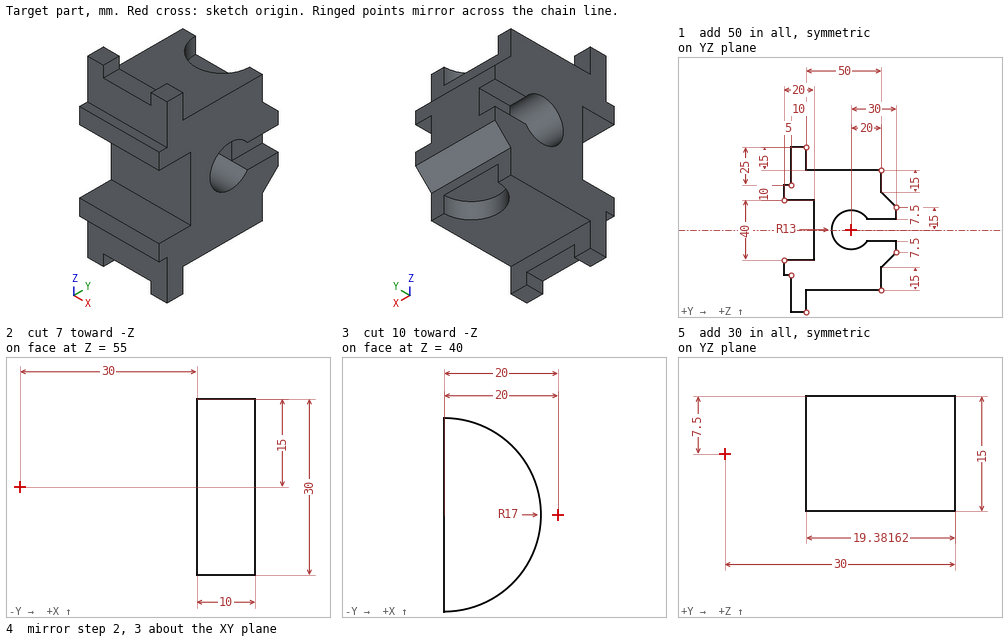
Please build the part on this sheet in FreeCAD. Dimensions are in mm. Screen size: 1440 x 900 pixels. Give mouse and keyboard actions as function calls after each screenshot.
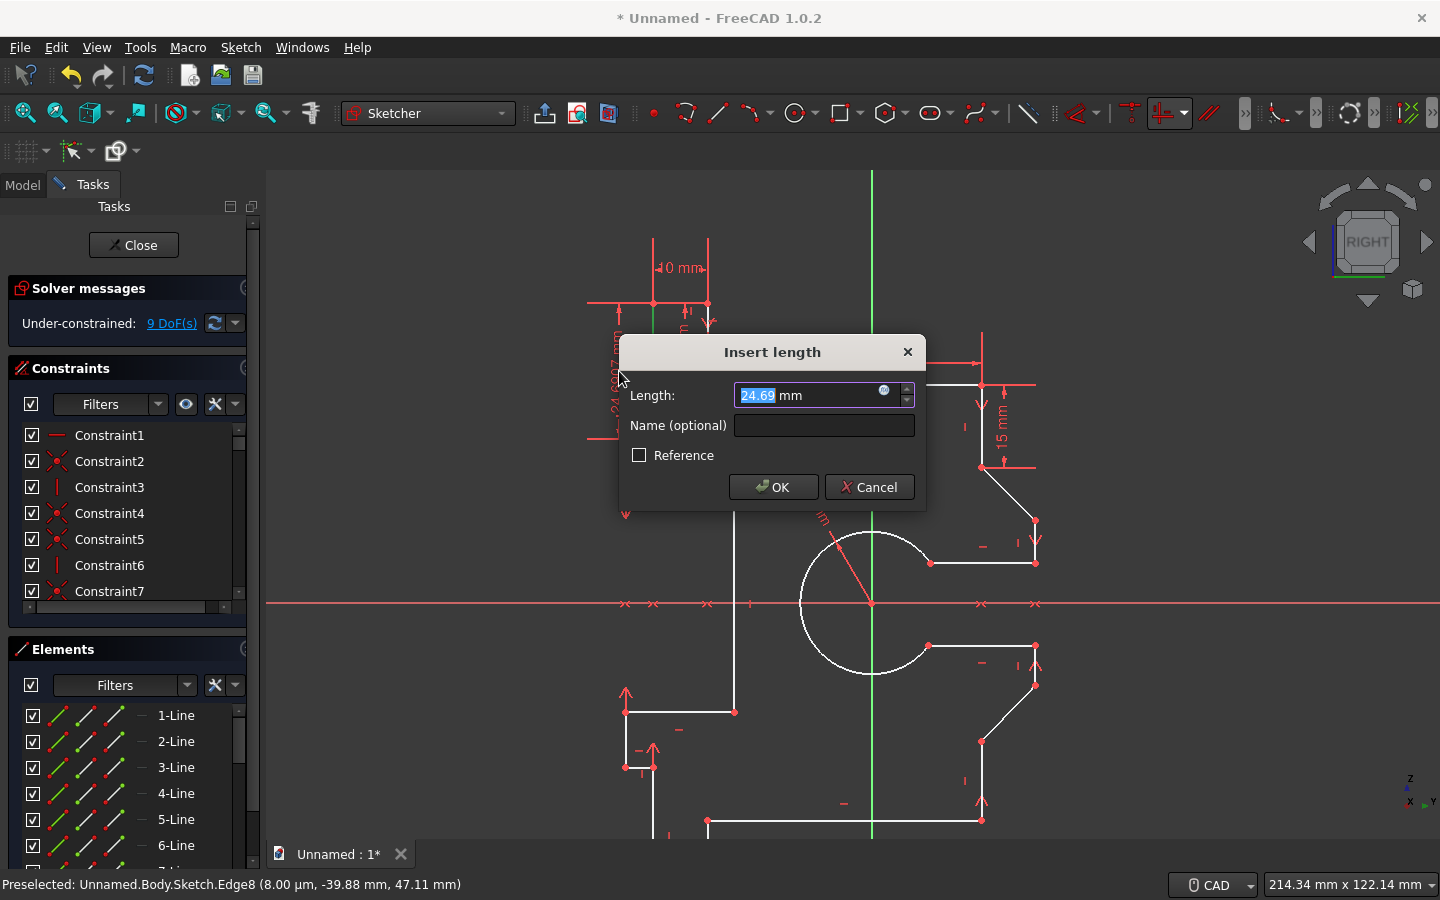
text(25)
key(Return)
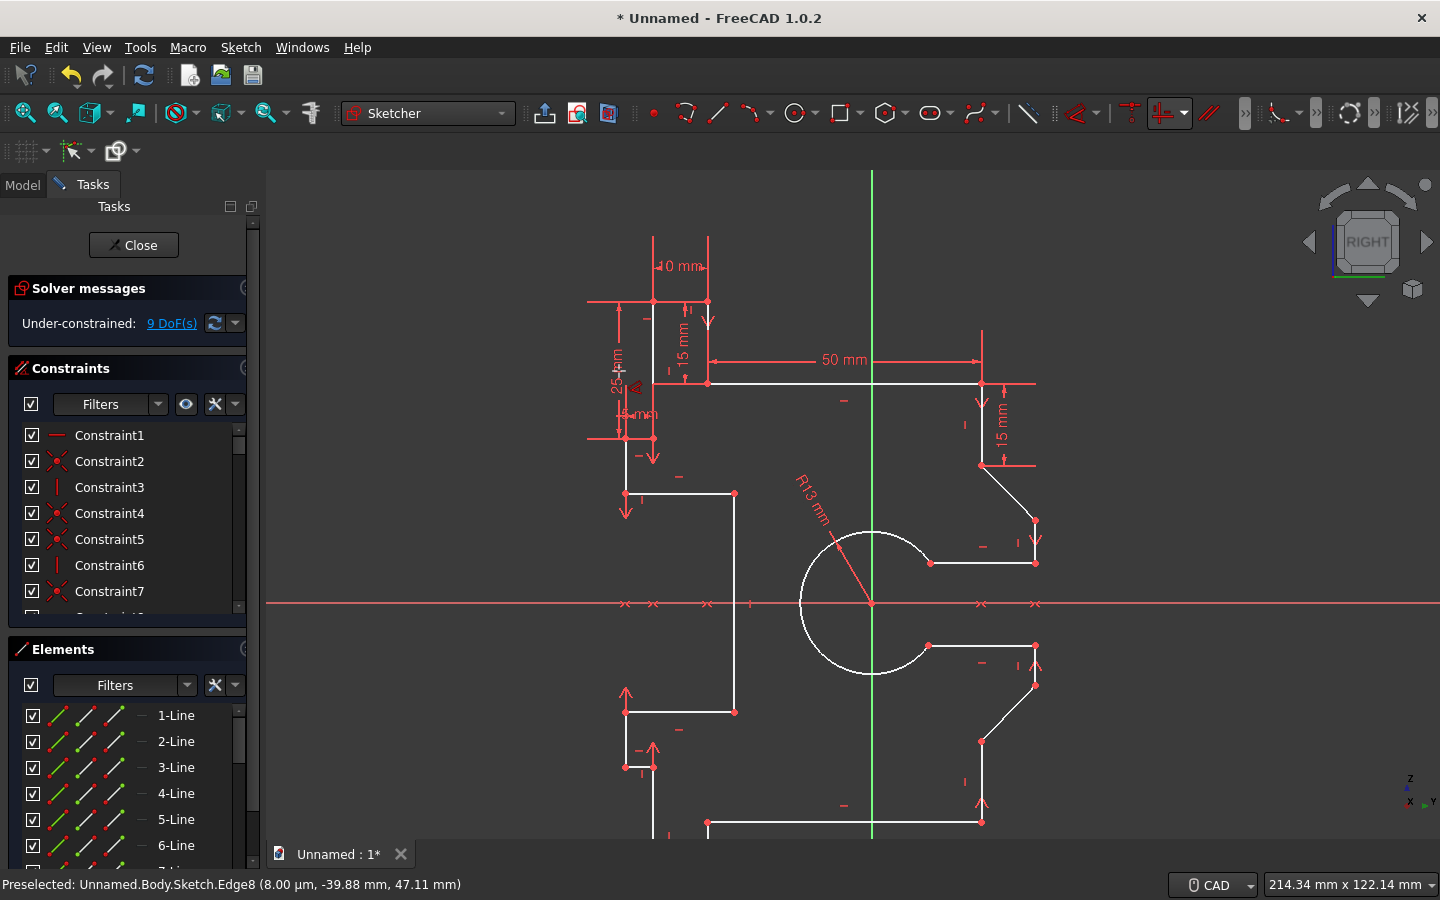
click(626, 455)
click(592, 466)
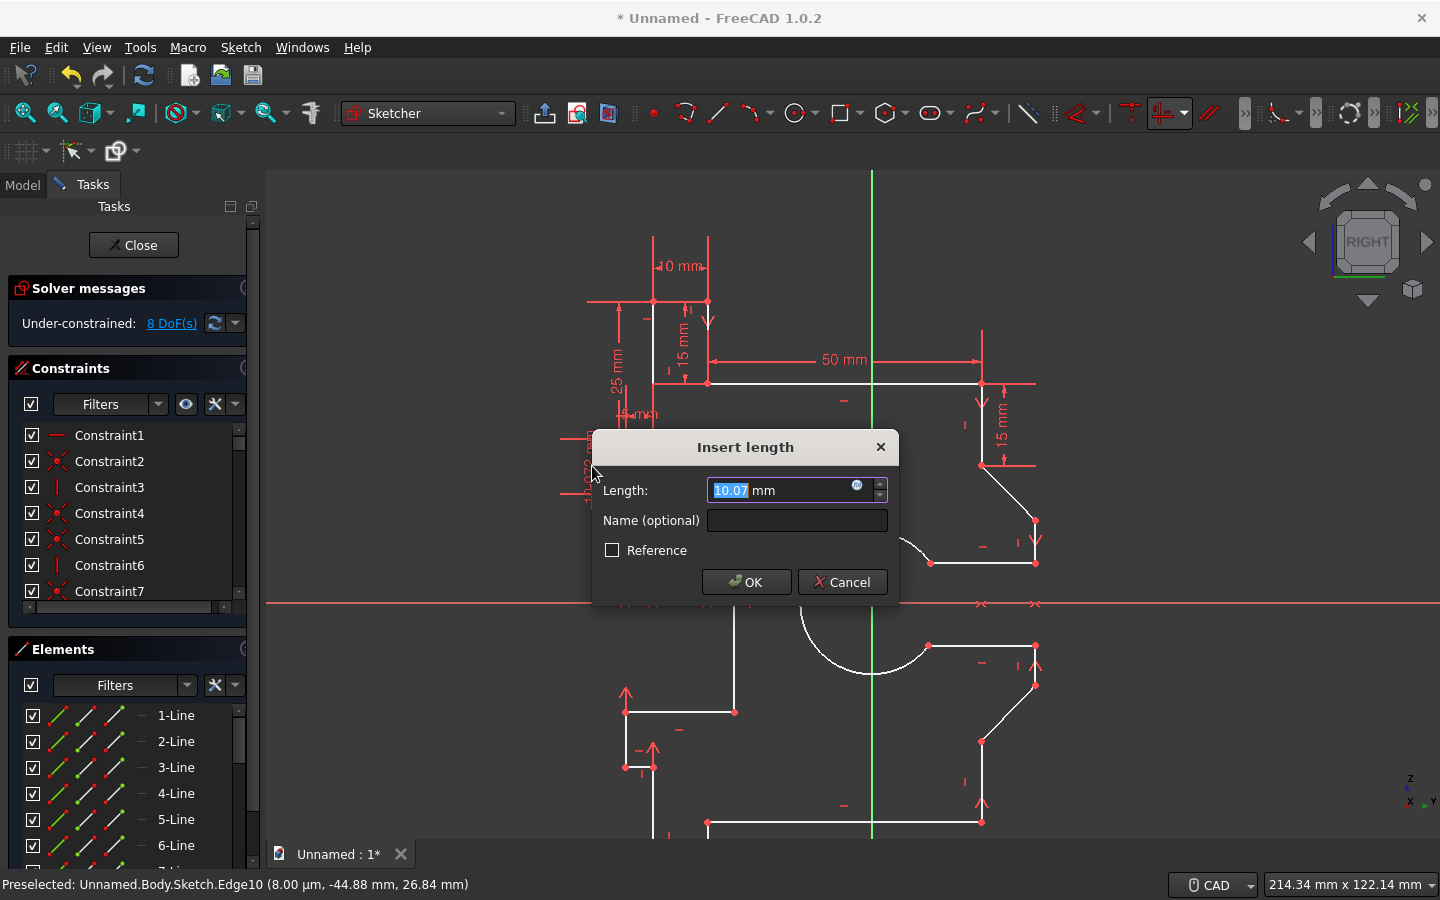
text(10)
key(Return)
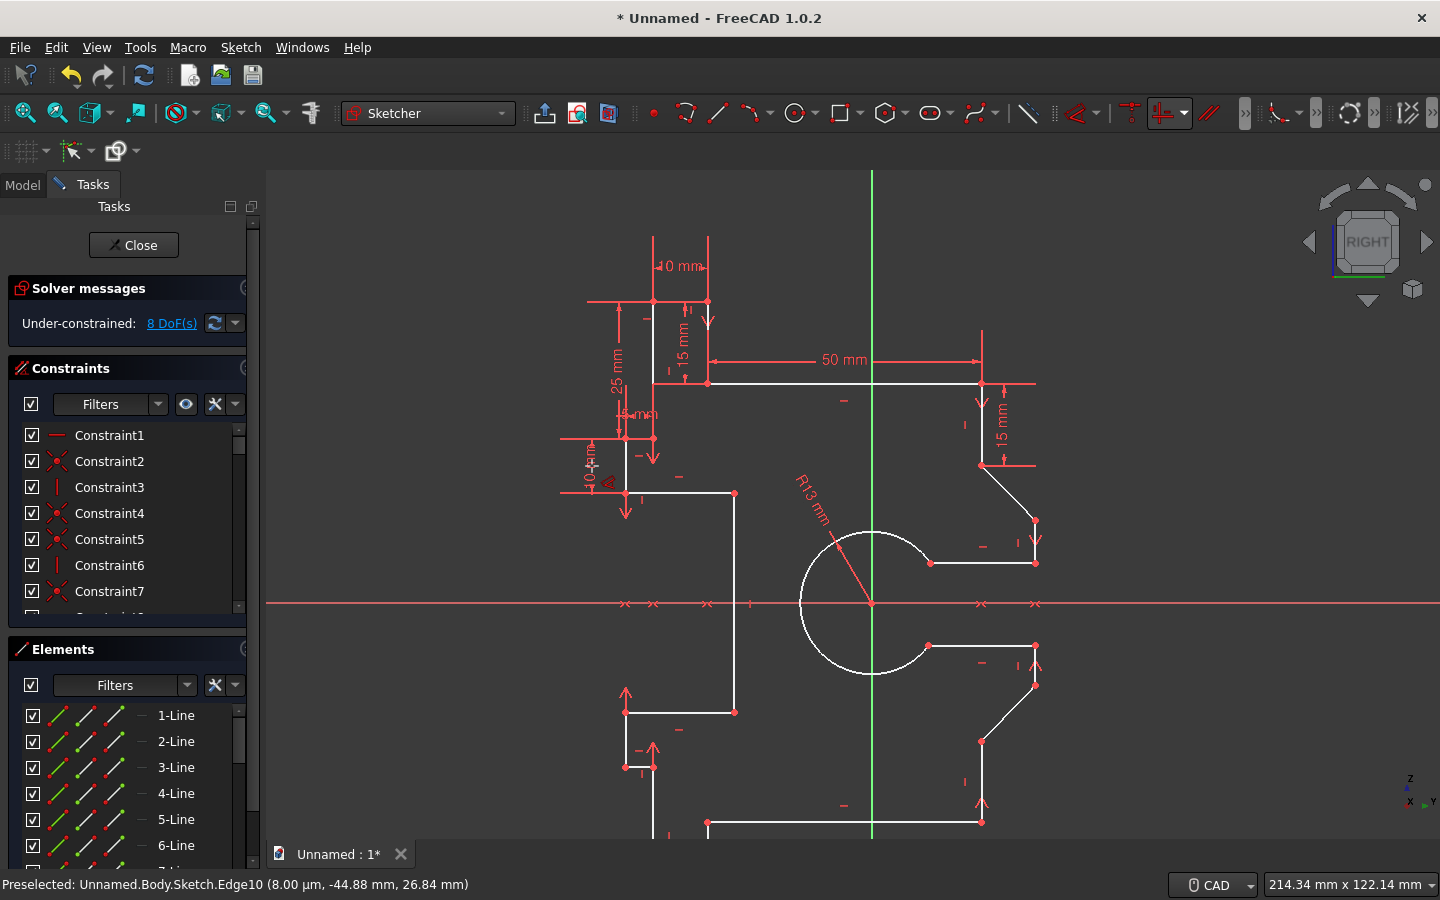
click(658, 493)
click(680, 459)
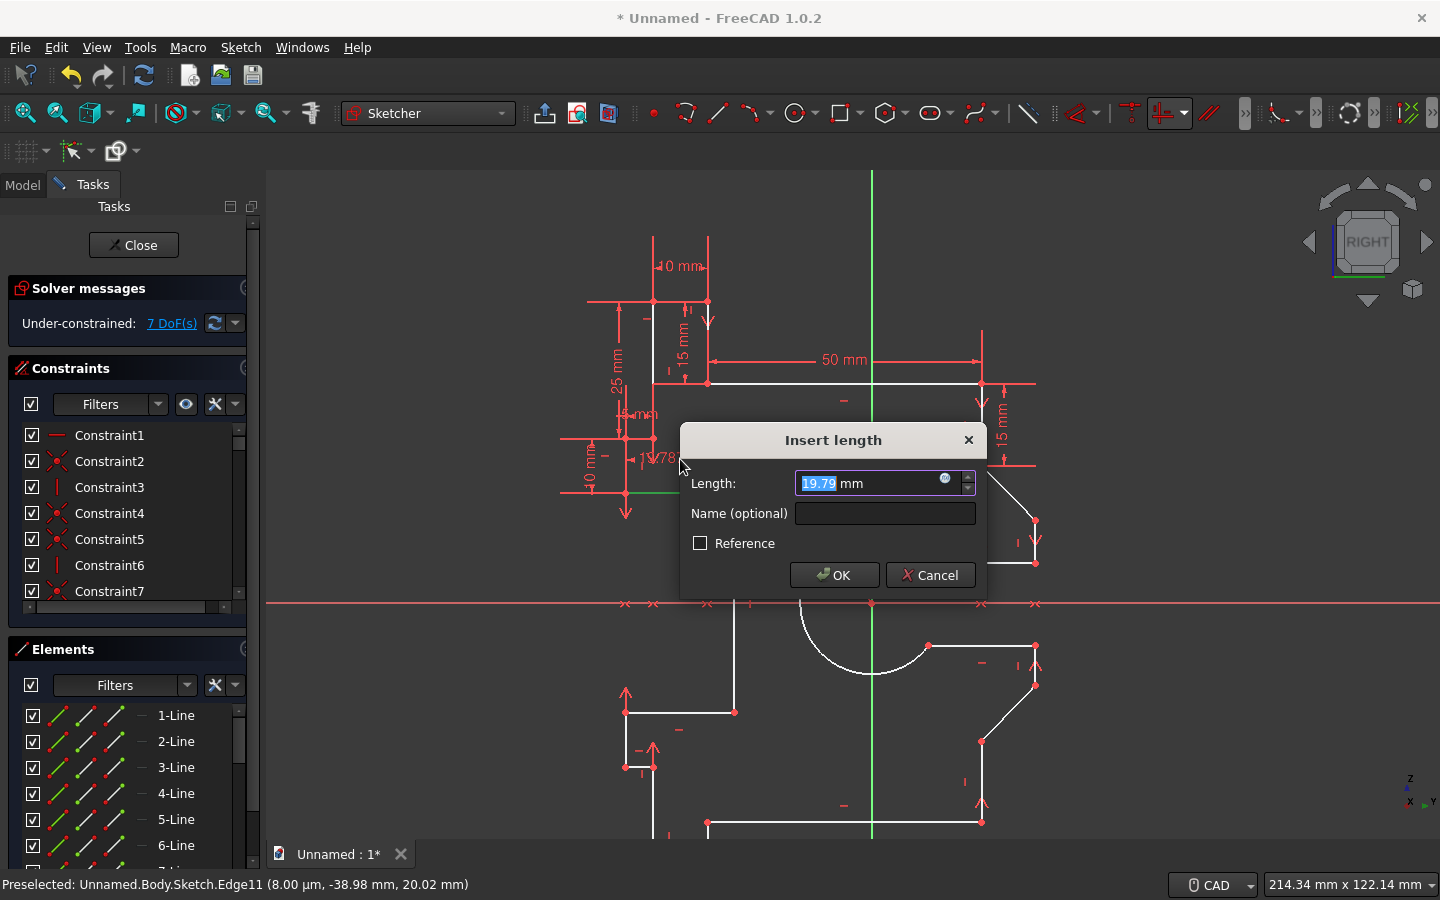
text(20)
key(Return)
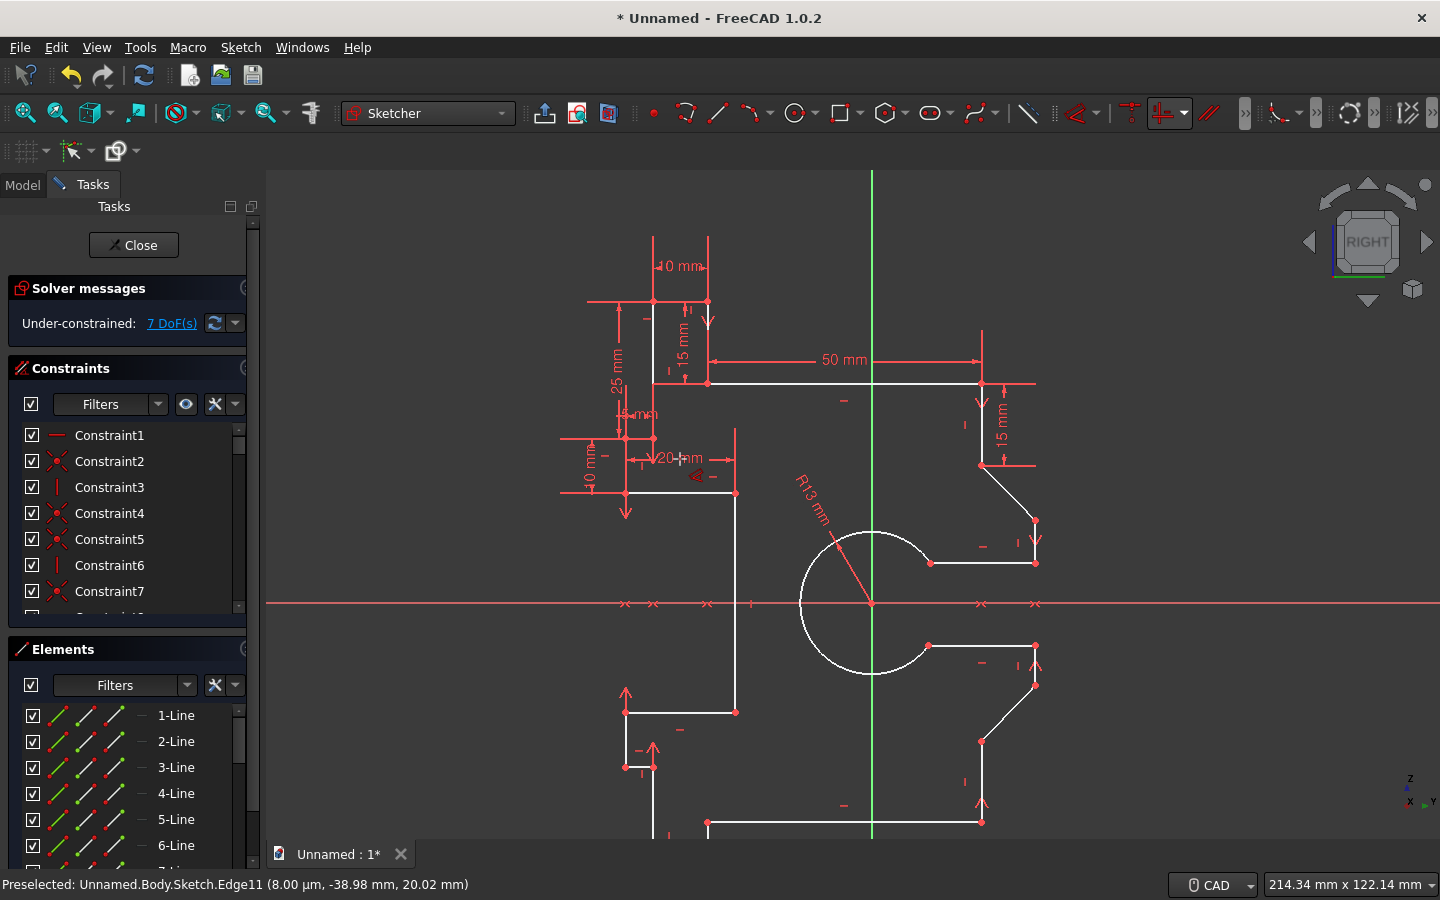
click(735, 559)
click(701, 553)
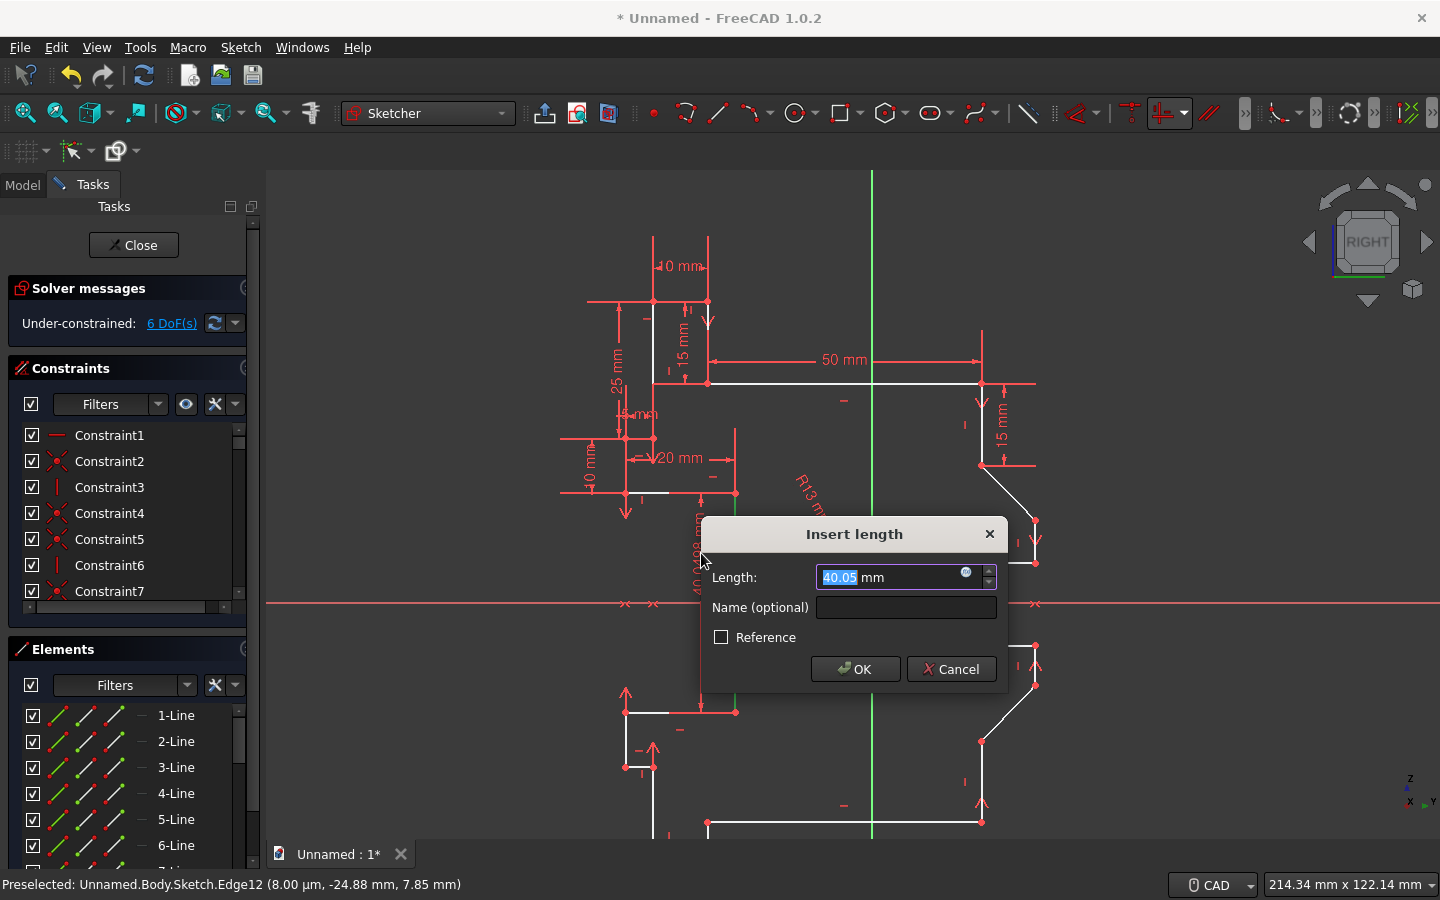
text(40)
key(Return)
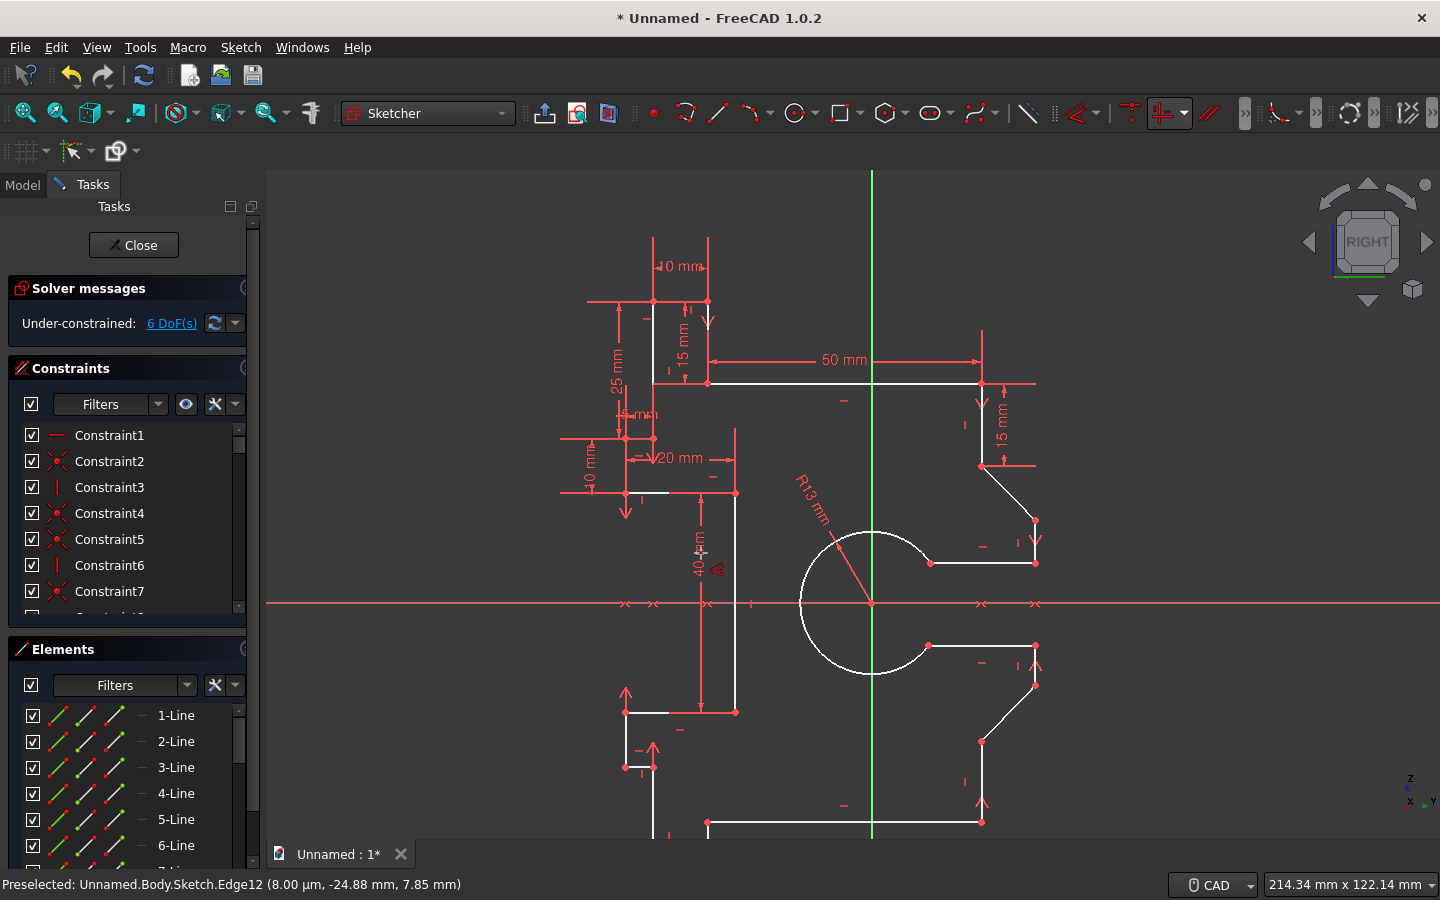
click(982, 798)
click(1016, 776)